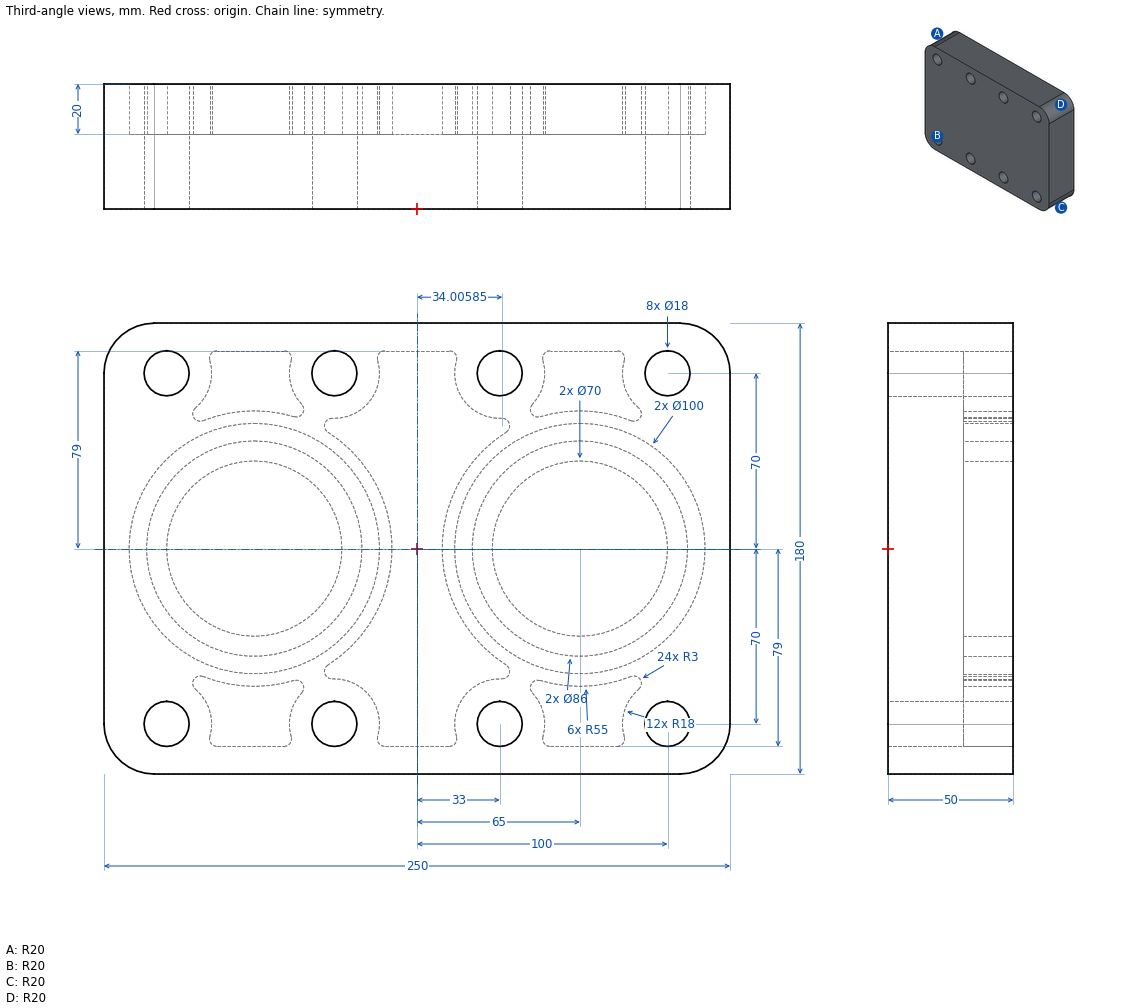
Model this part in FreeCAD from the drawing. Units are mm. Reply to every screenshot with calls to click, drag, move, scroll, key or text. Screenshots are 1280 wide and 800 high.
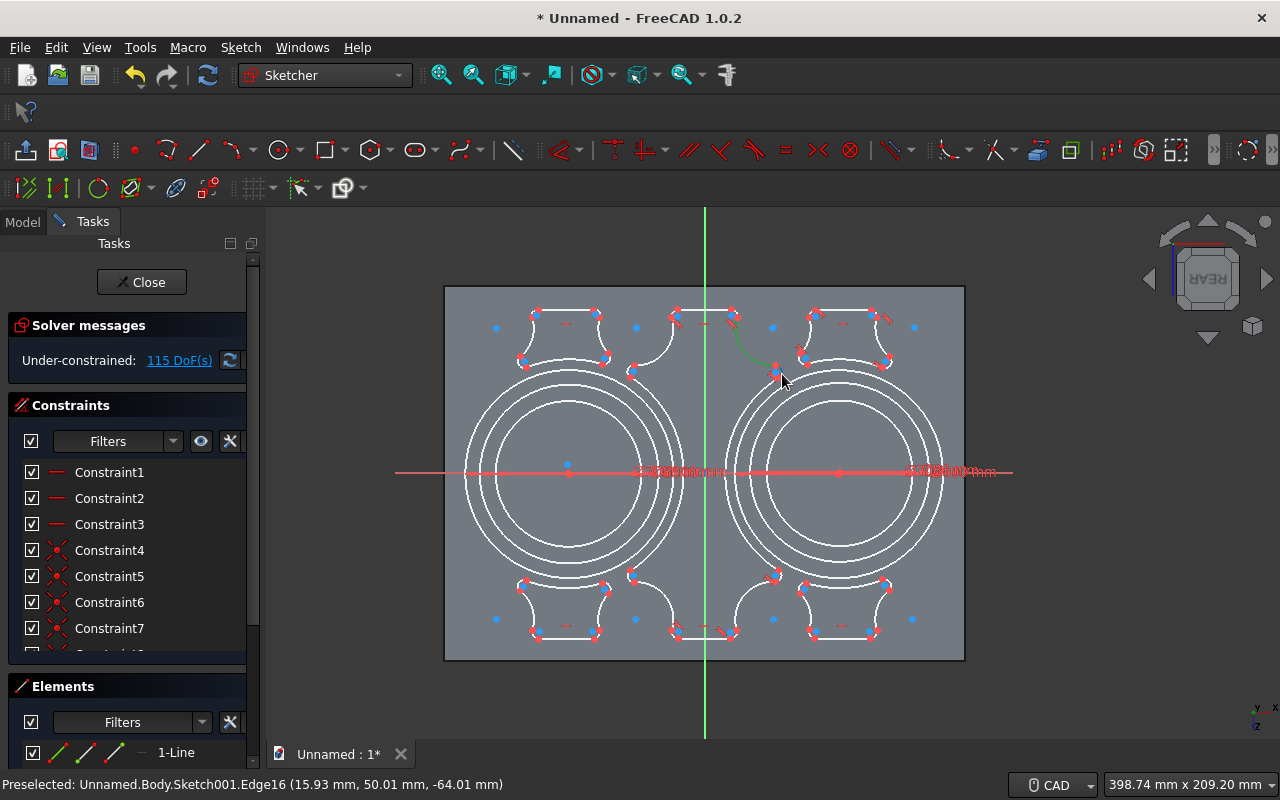
scroll(737, 312, up, 5)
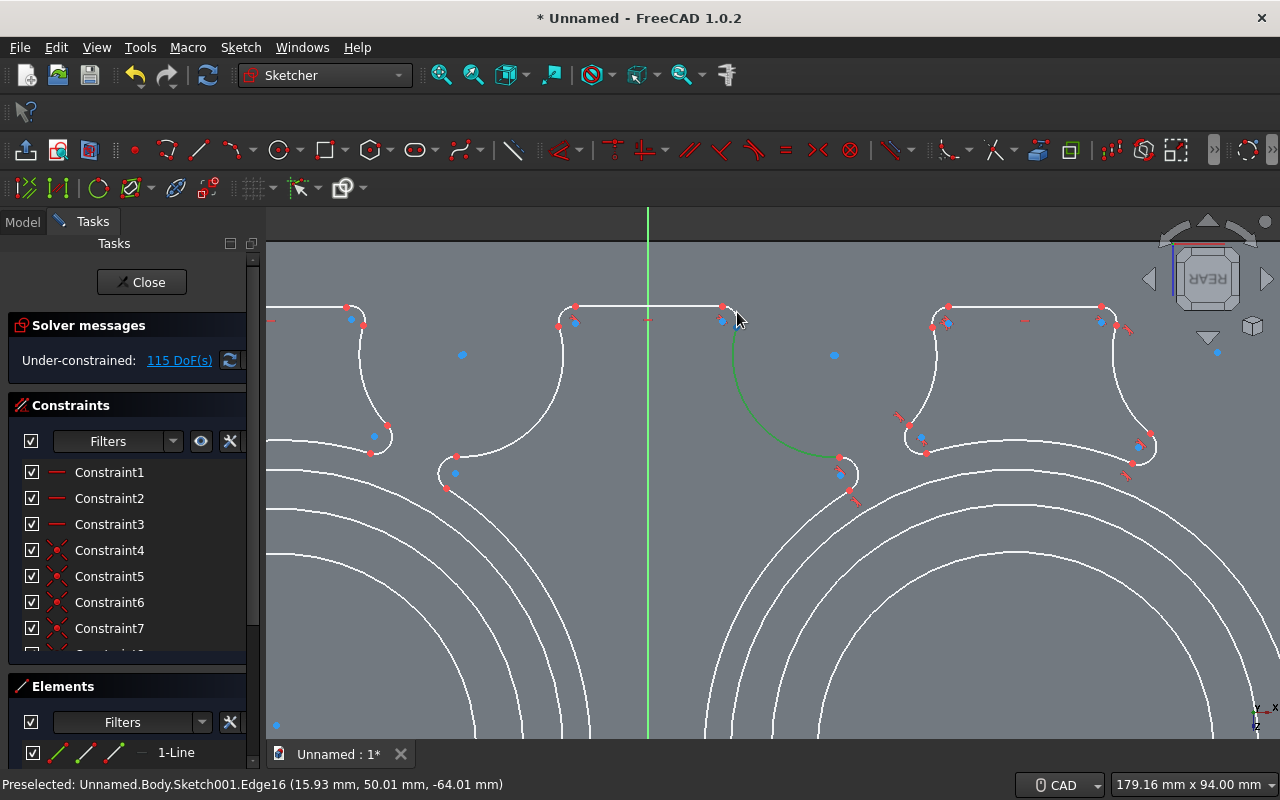
click(735, 313)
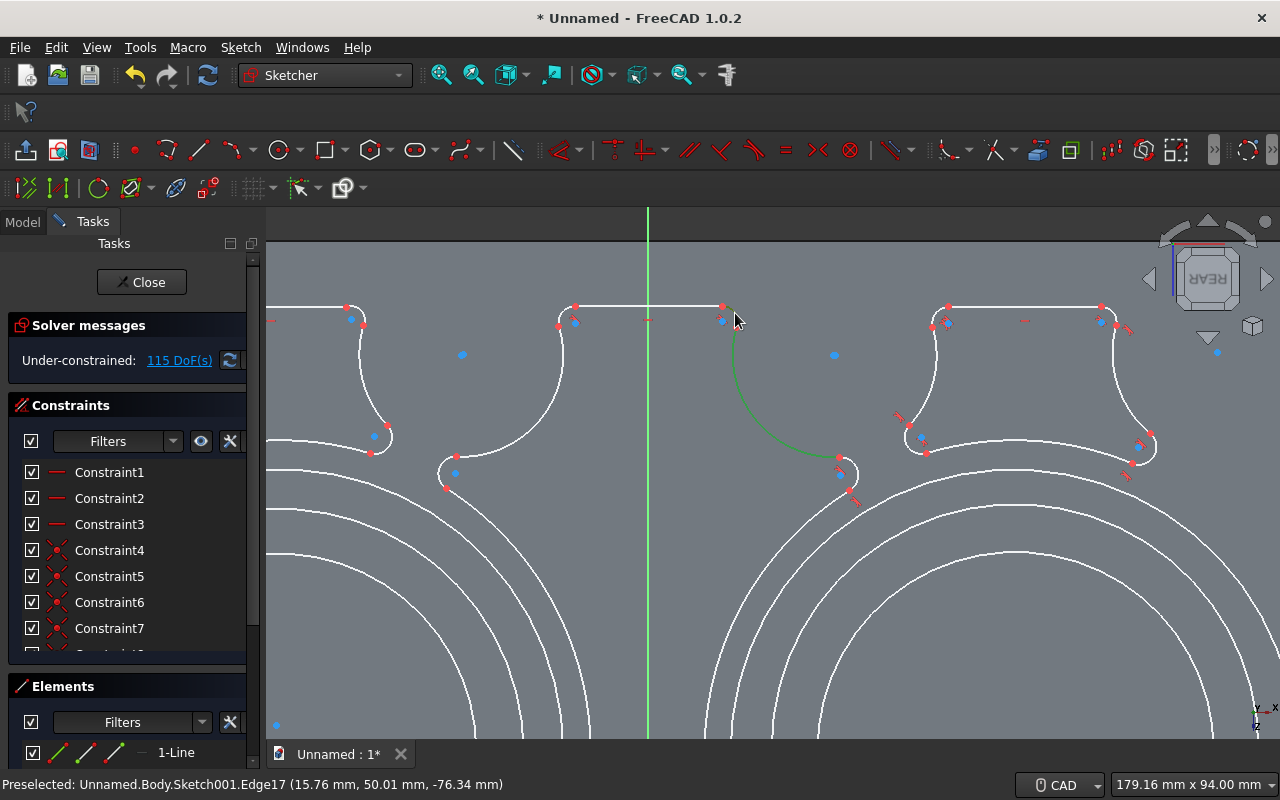
click(754, 150)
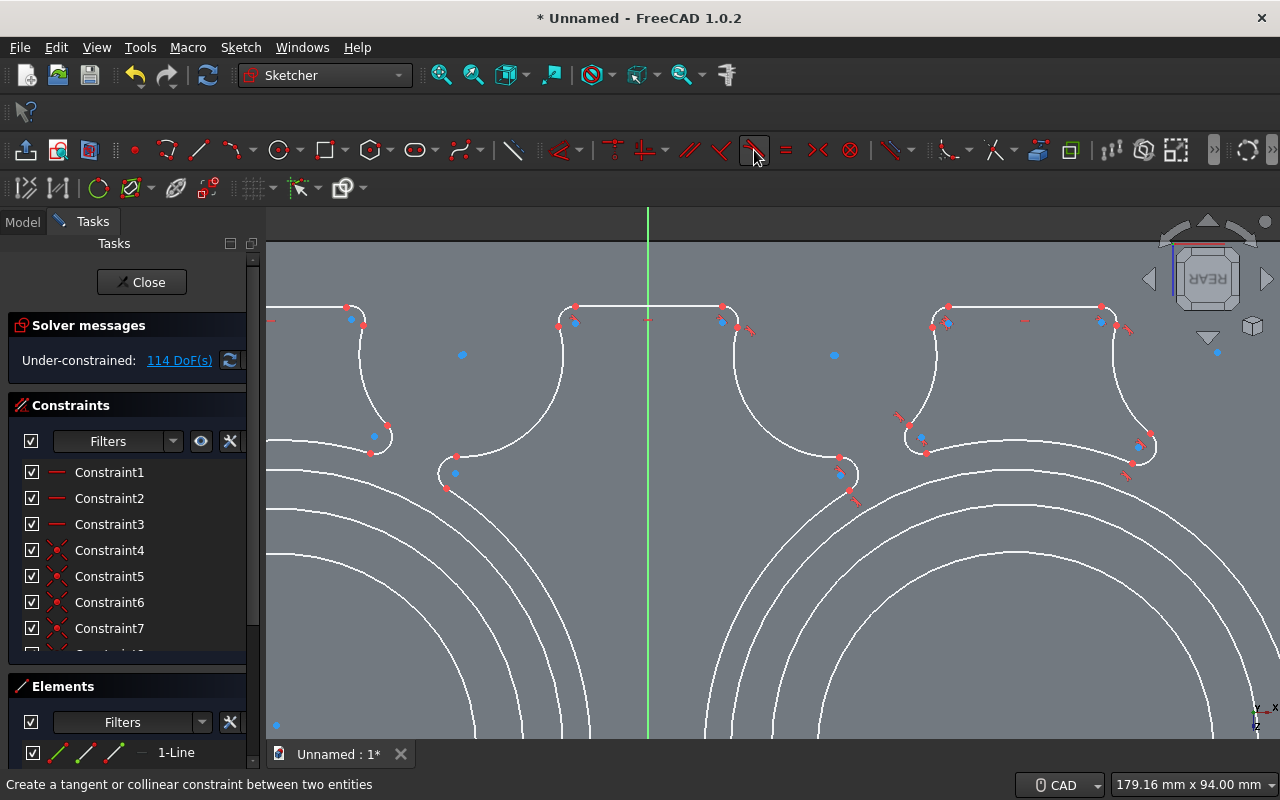
click(562, 312)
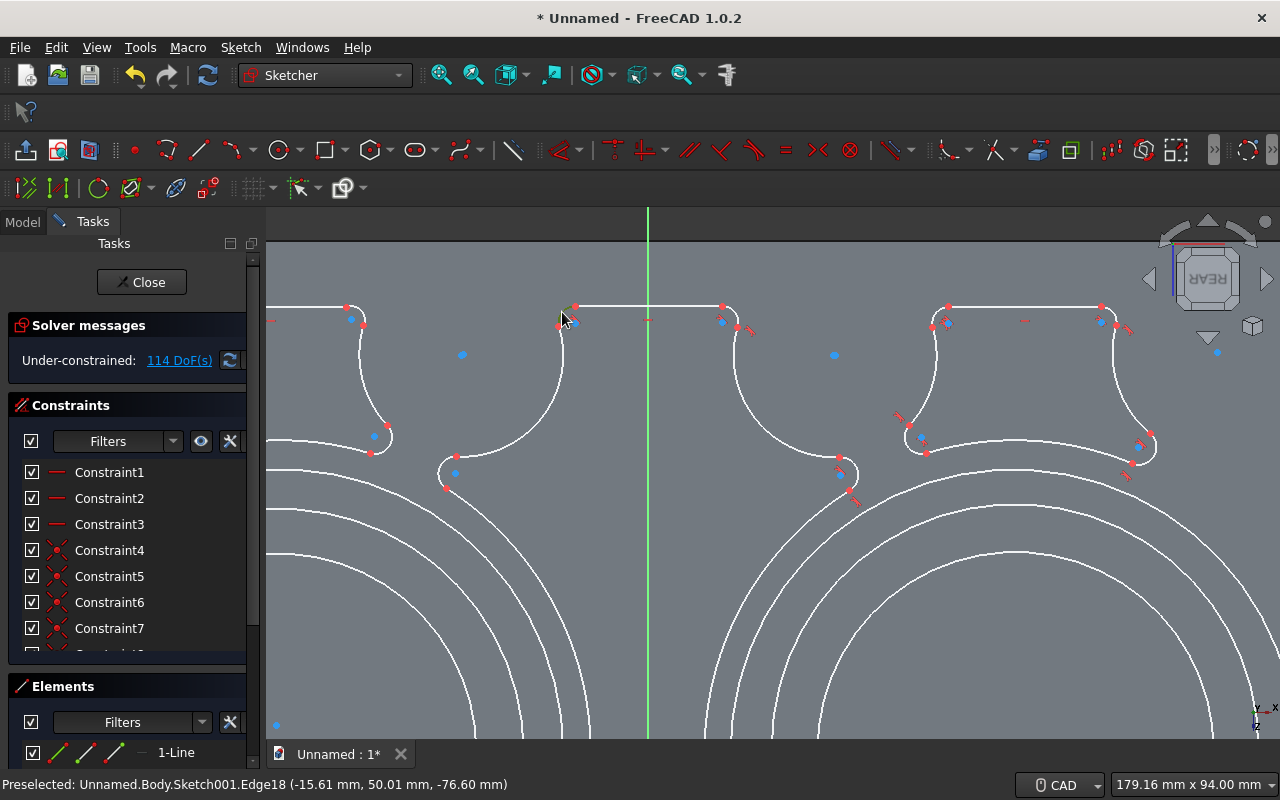
click(513, 443)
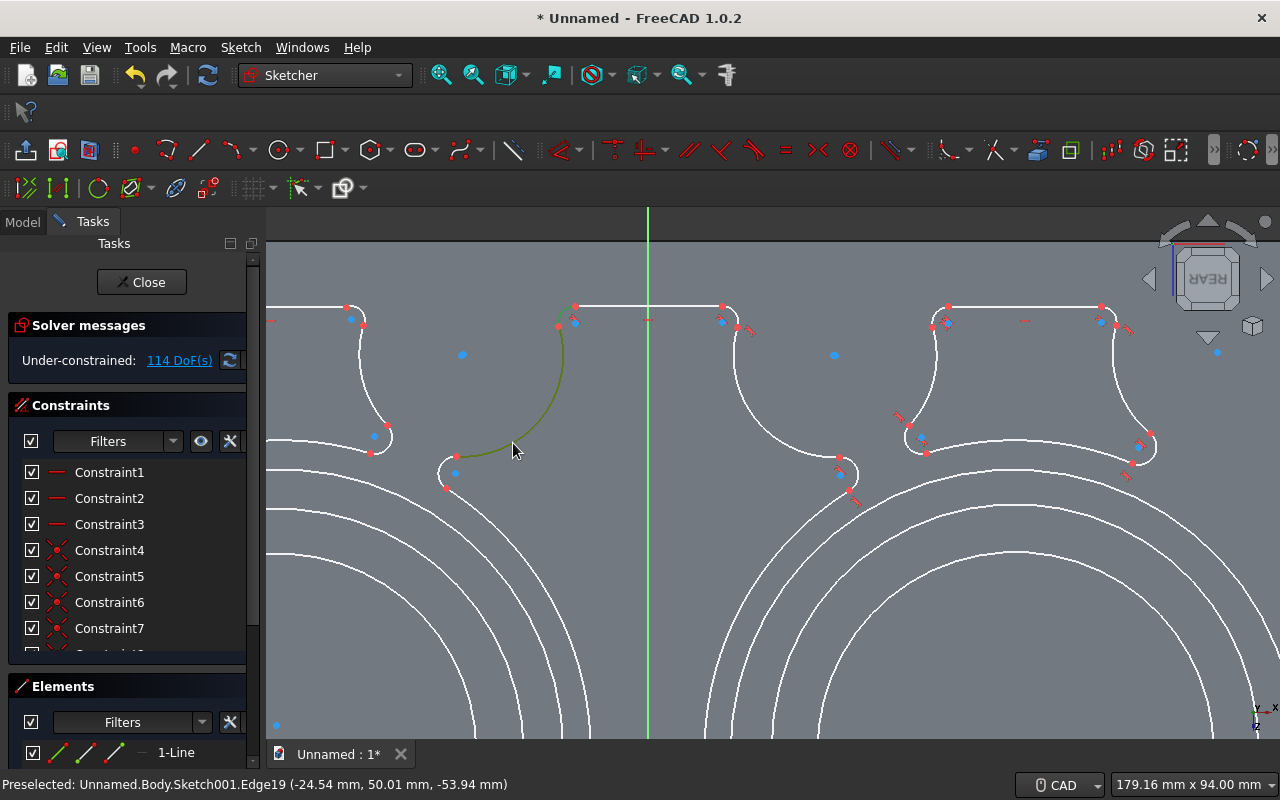
click(754, 150)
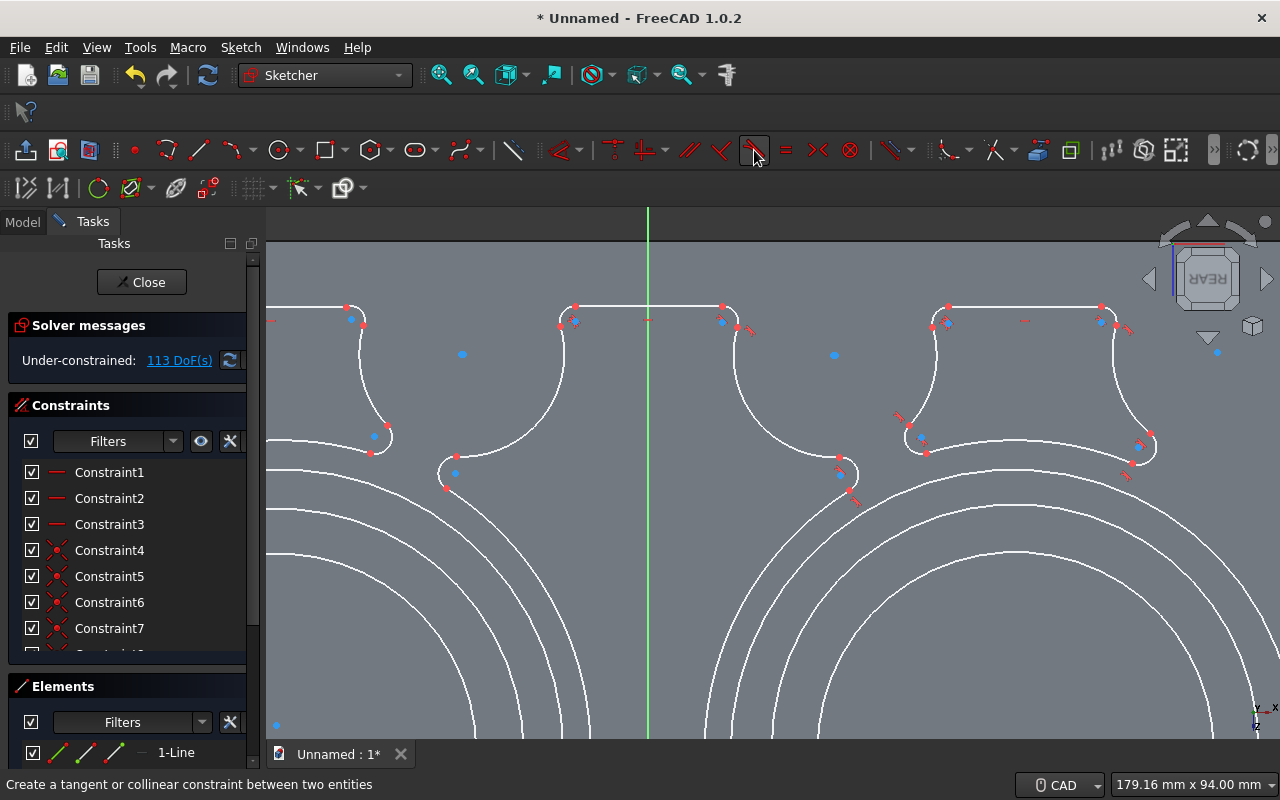
click(513, 443)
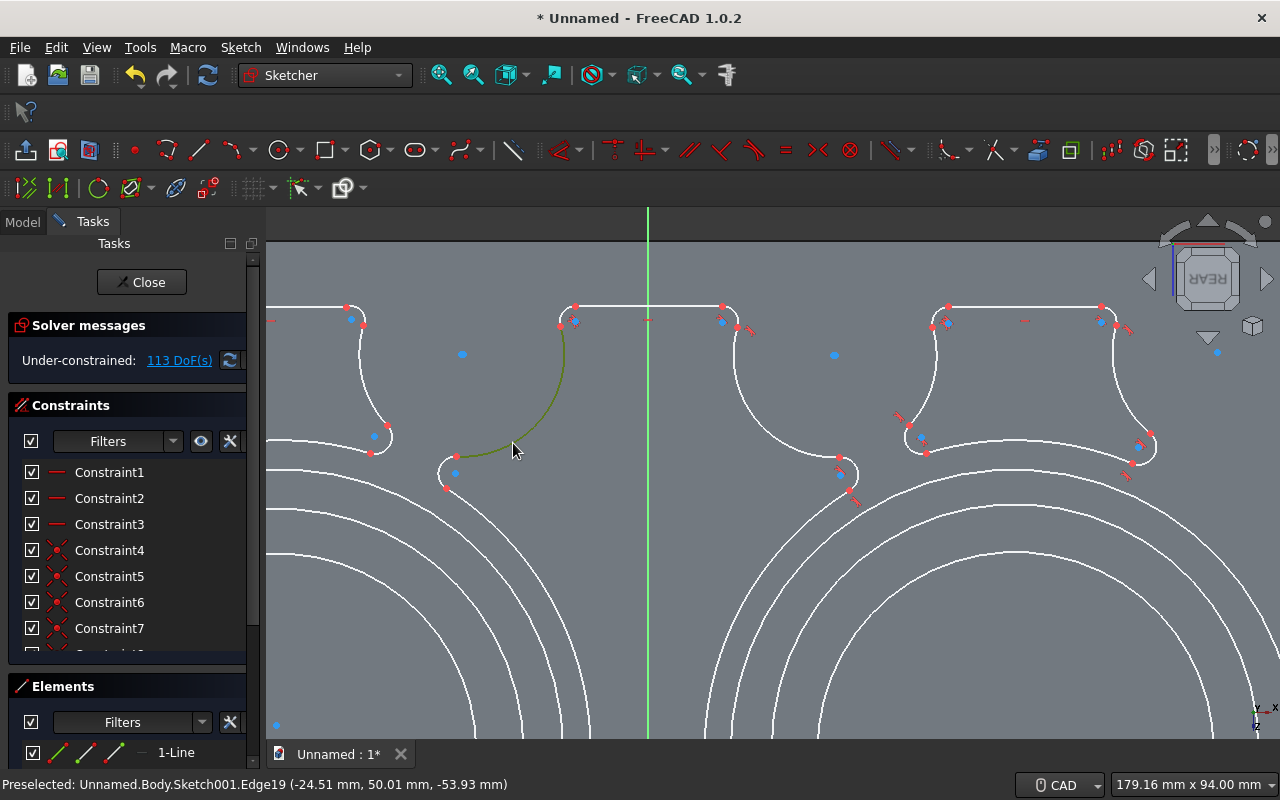
click(444, 461)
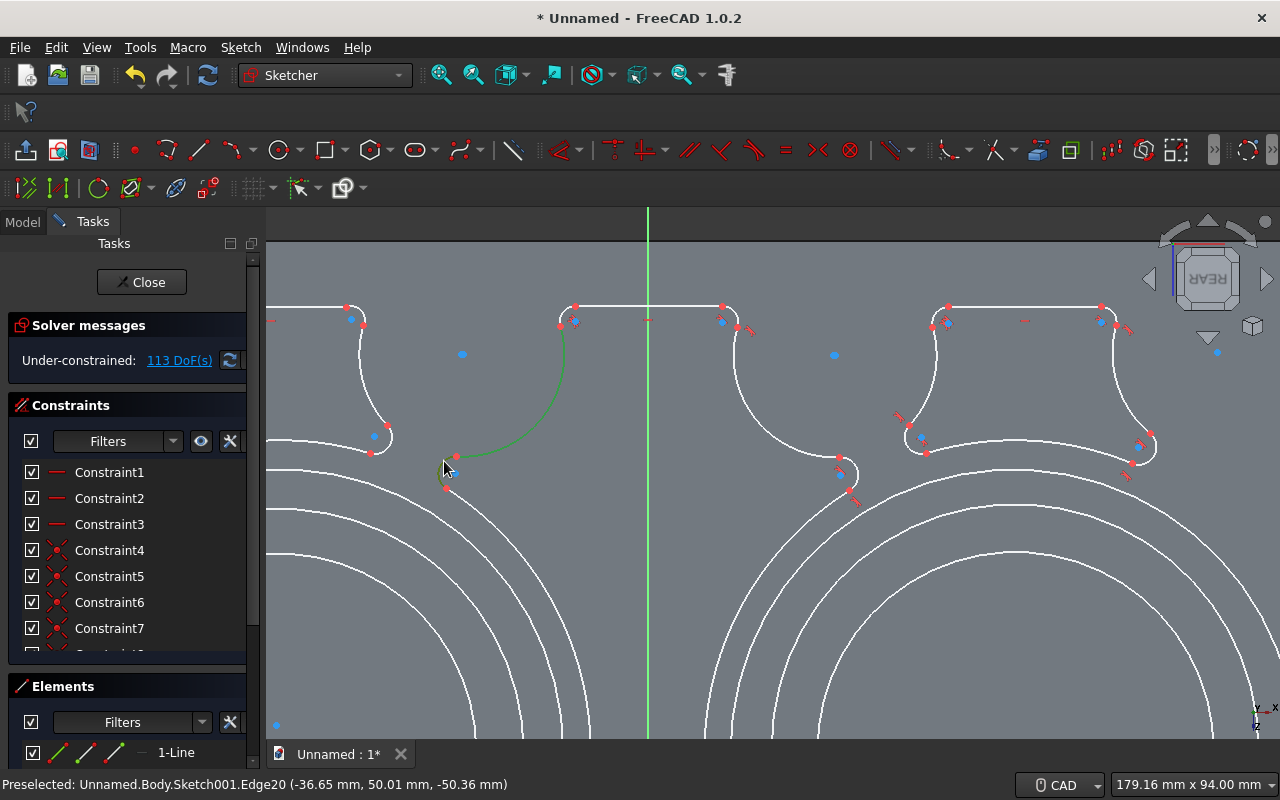
click(754, 150)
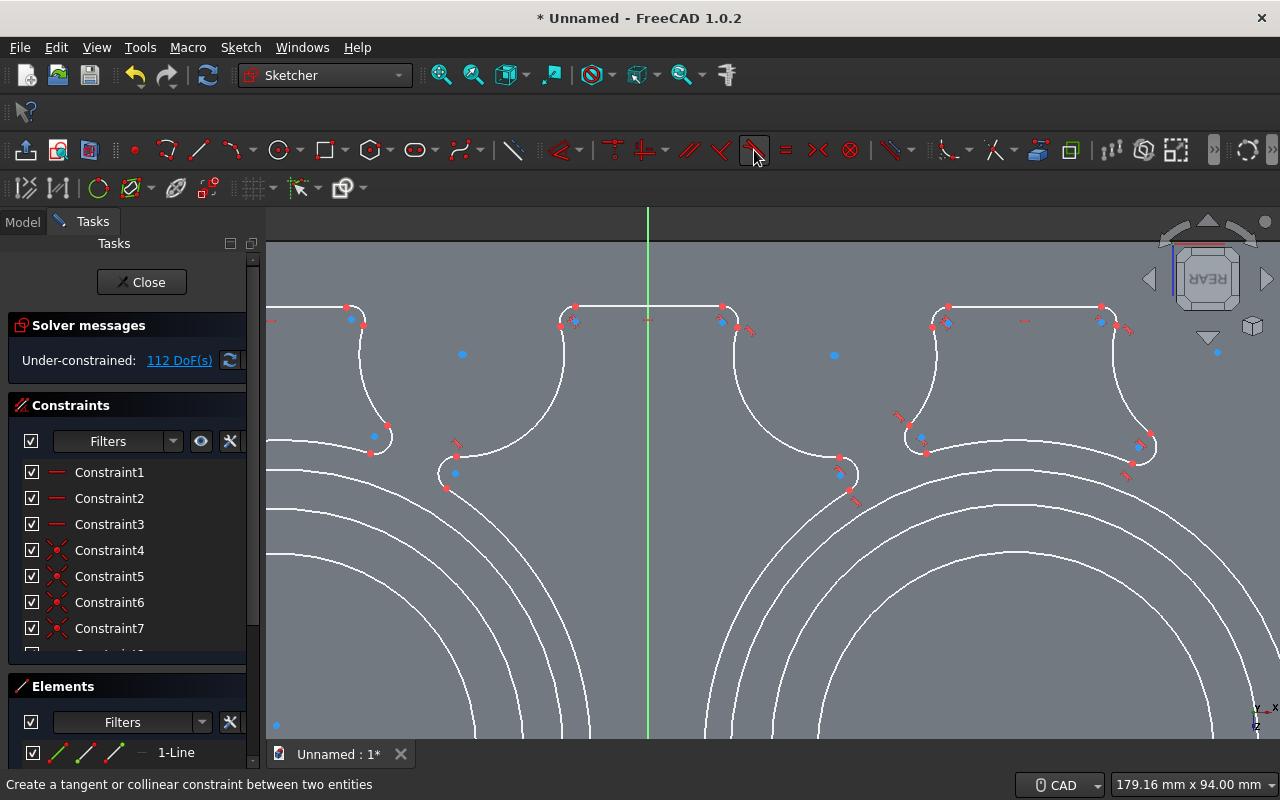
click(444, 461)